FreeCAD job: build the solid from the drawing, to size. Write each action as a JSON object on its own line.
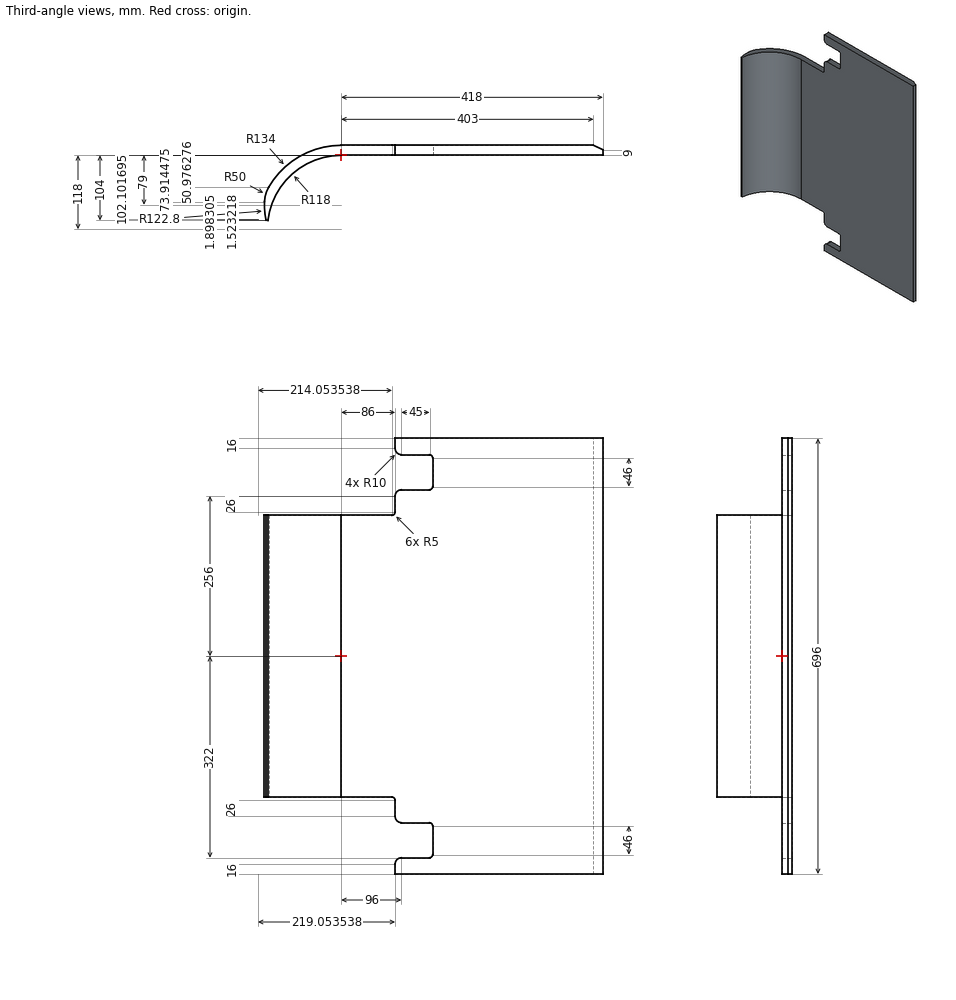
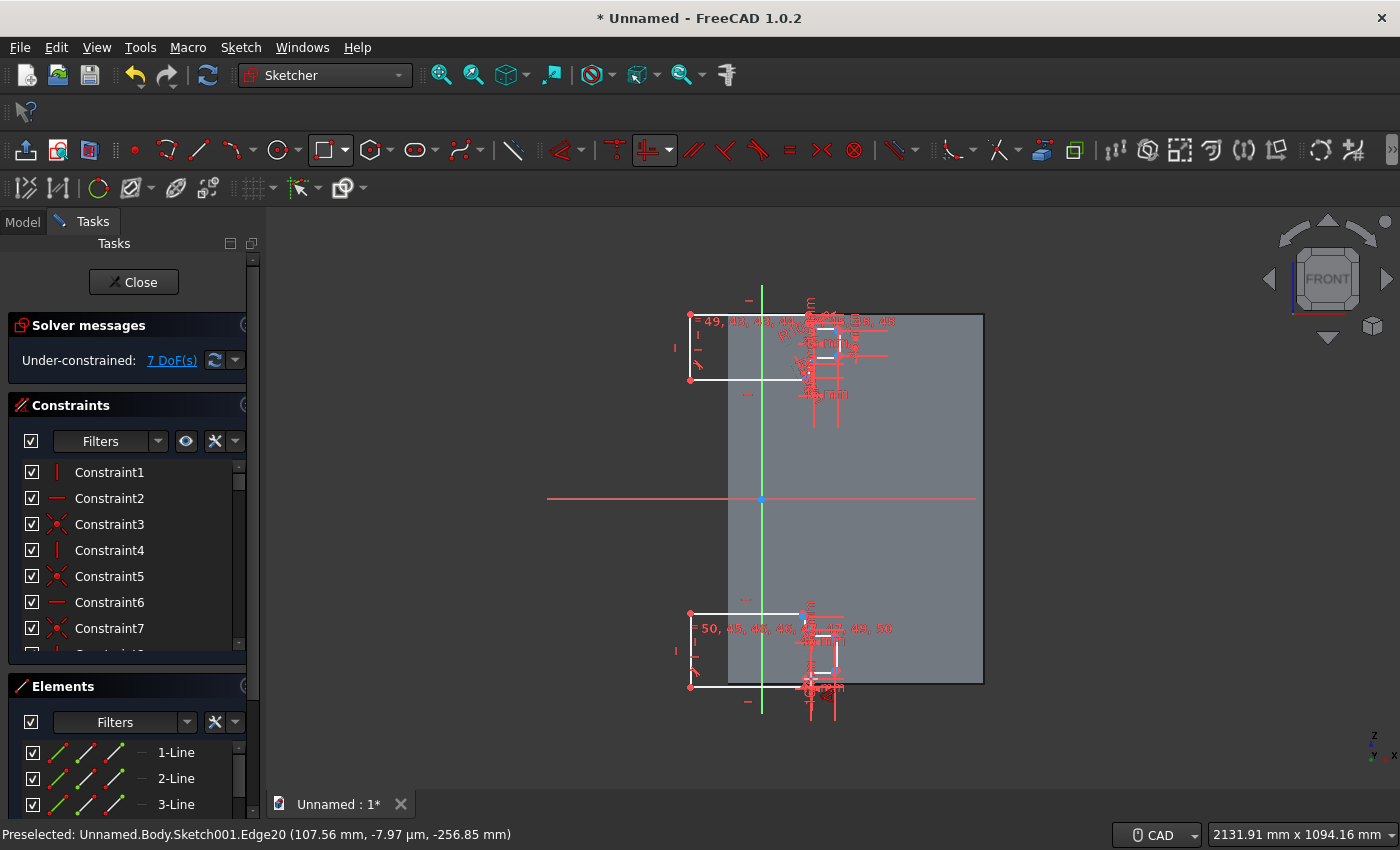
{"action": "scroll", "coordinate": [837, 648], "scroll_direction": "up", "scroll_amount": 3}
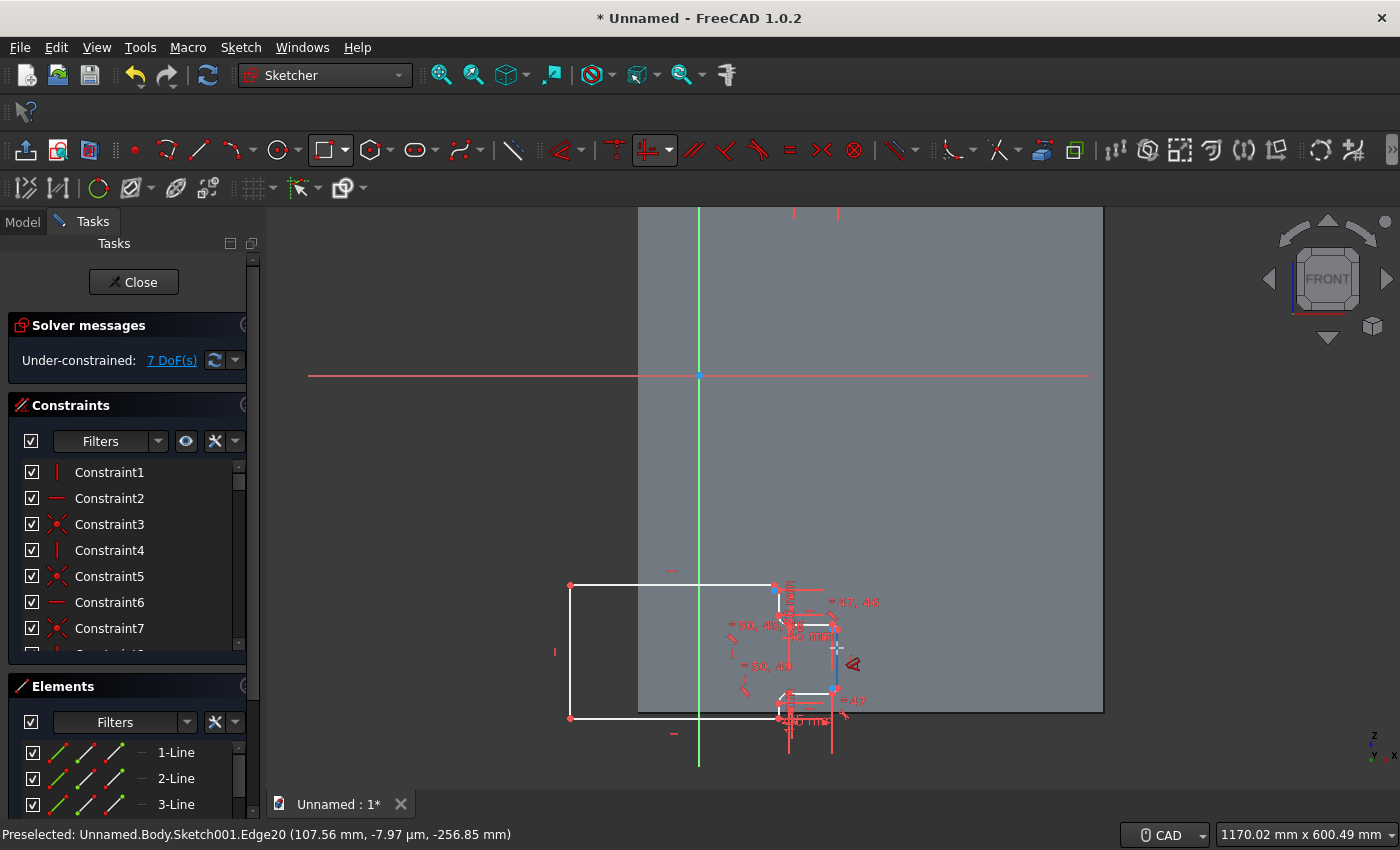
{"action": "left_click", "coordinate": [837, 647]}
{"action": "left_click", "coordinate": [871, 659]}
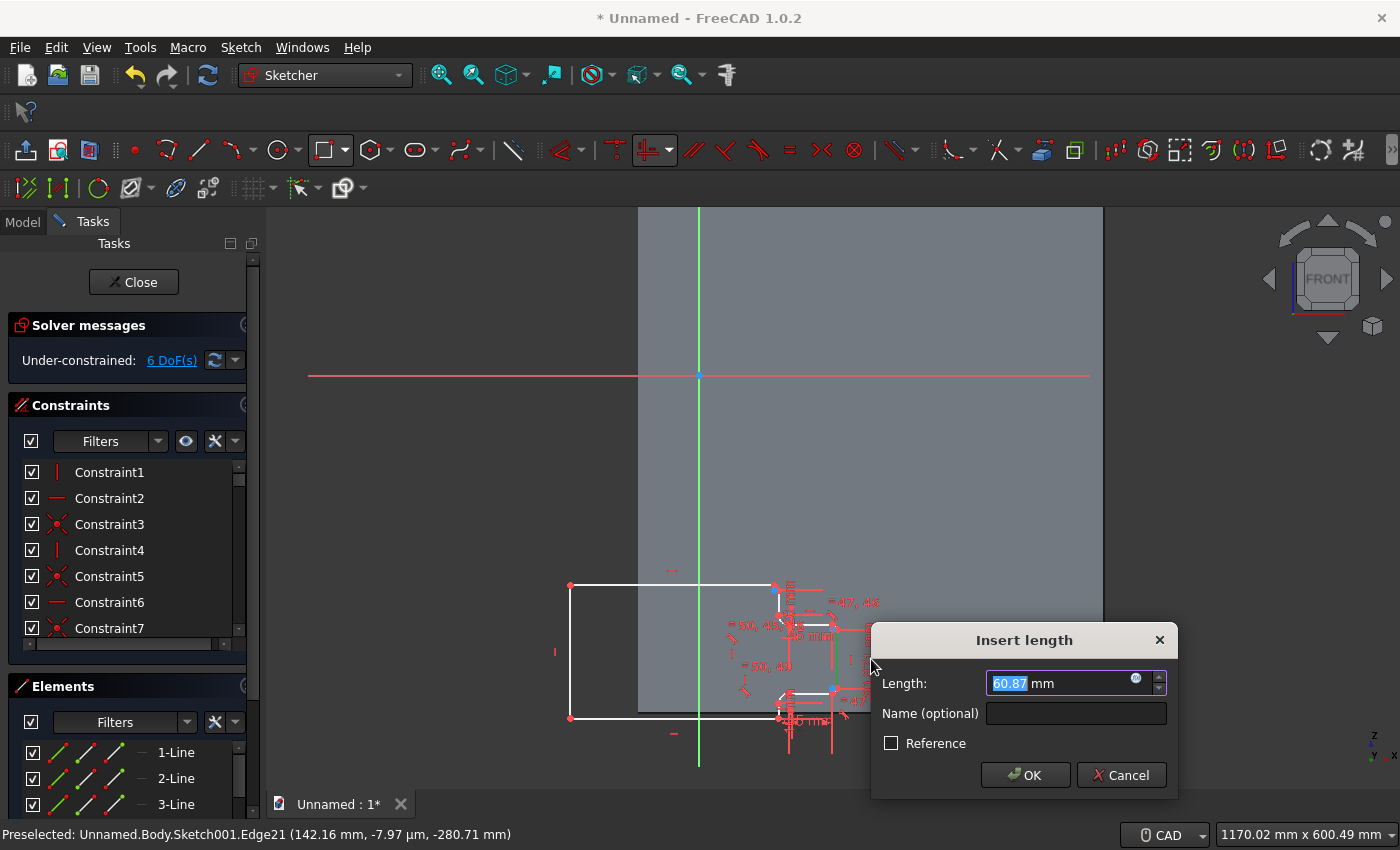
{"action": "type", "text": "46"}
{"action": "key", "text": "Return"}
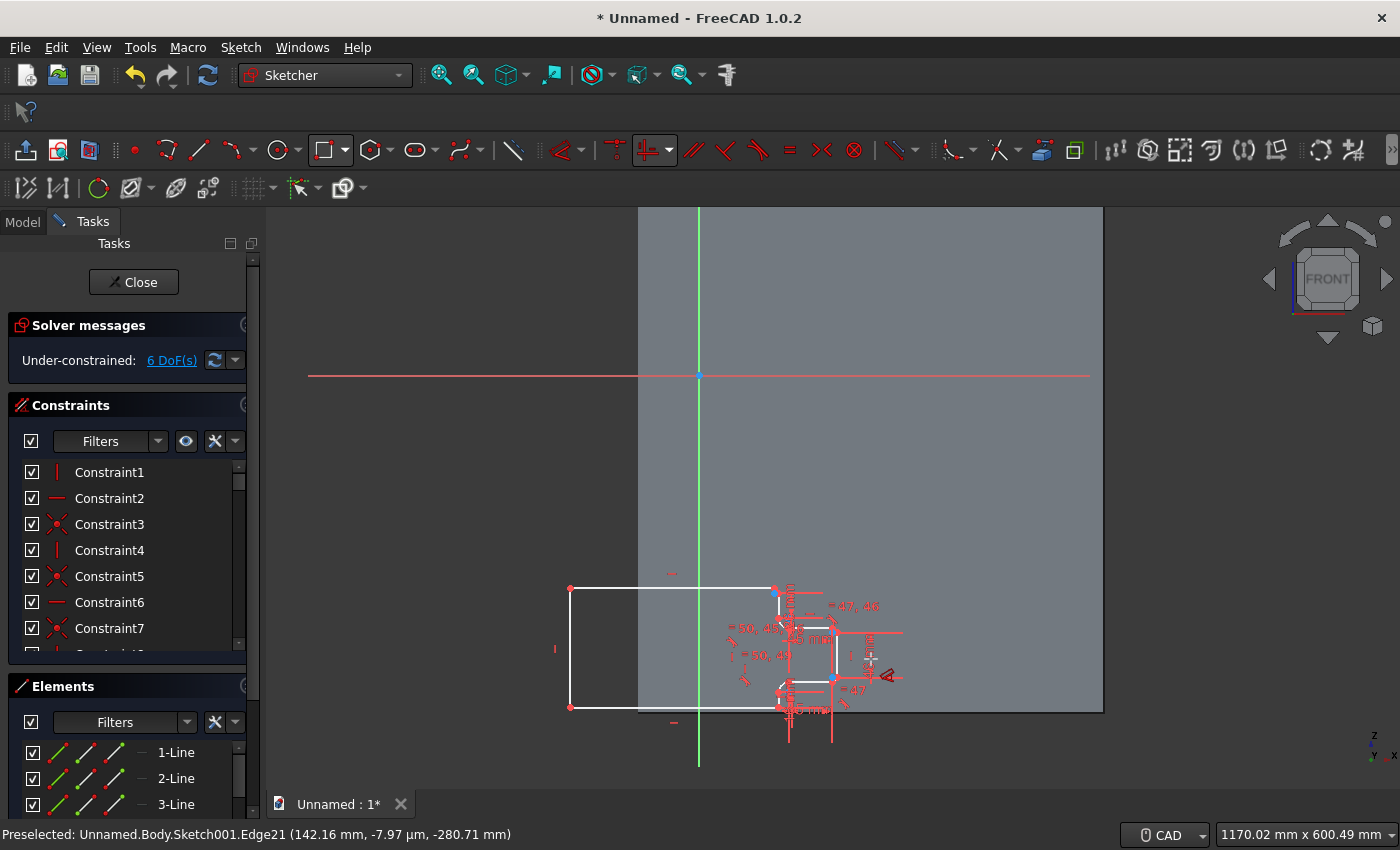
{"action": "scroll", "coordinate": [836, 646], "scroll_direction": "down", "scroll_amount": 3}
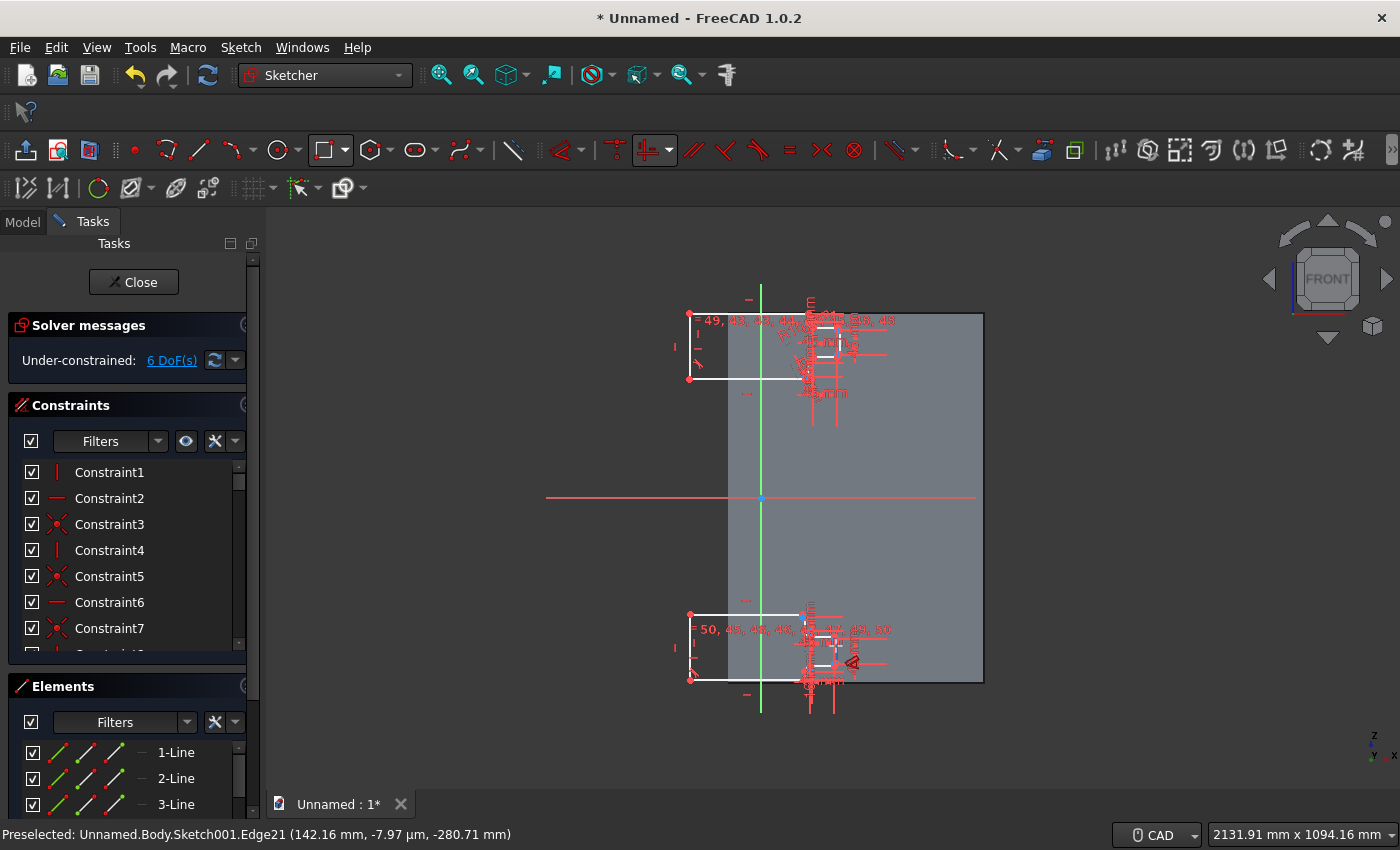
{"action": "scroll", "coordinate": [808, 363], "scroll_direction": "up", "scroll_amount": 5}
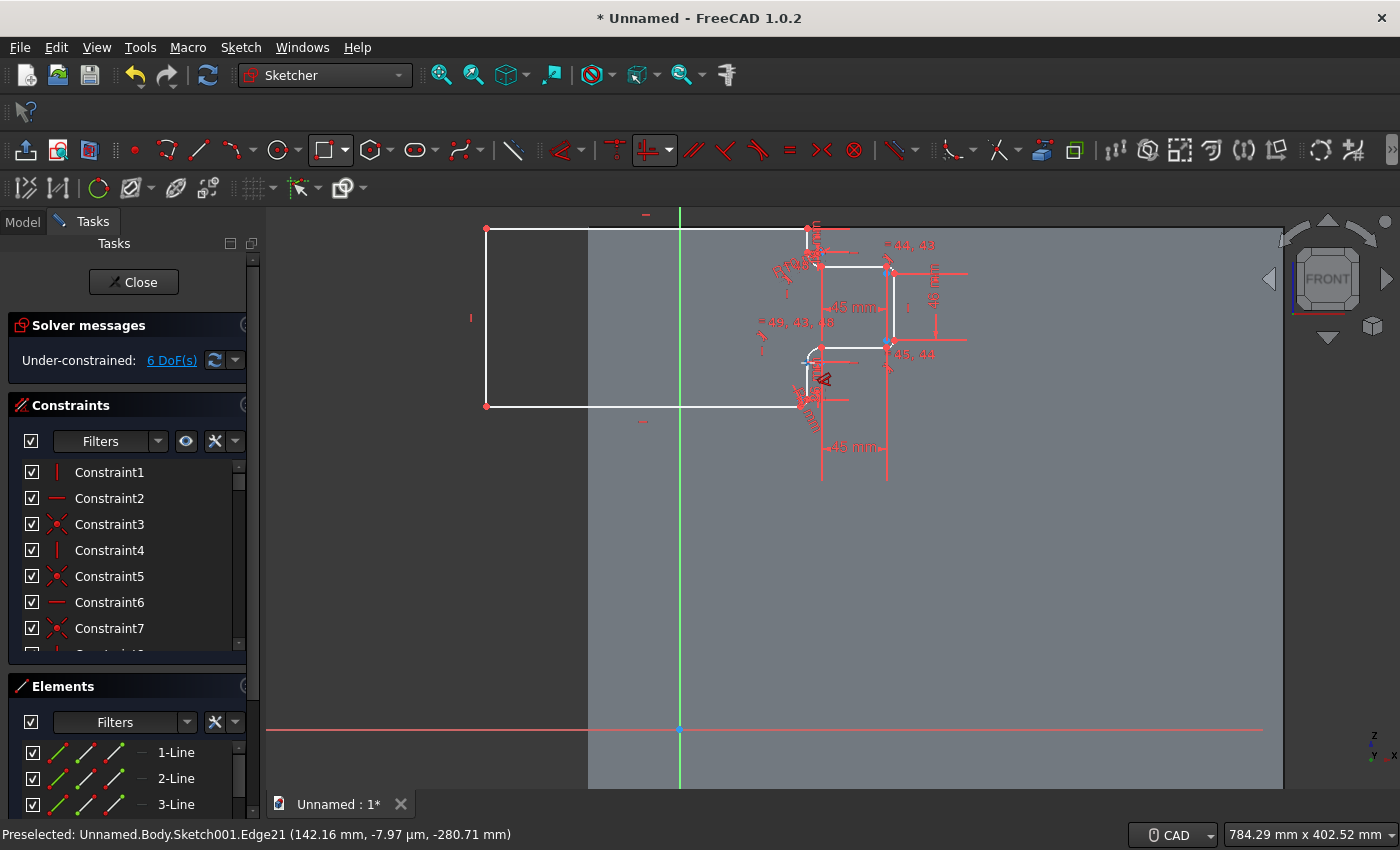
{"action": "left_click", "coordinate": [807, 362]}
{"action": "left_click", "coordinate": [744, 328]}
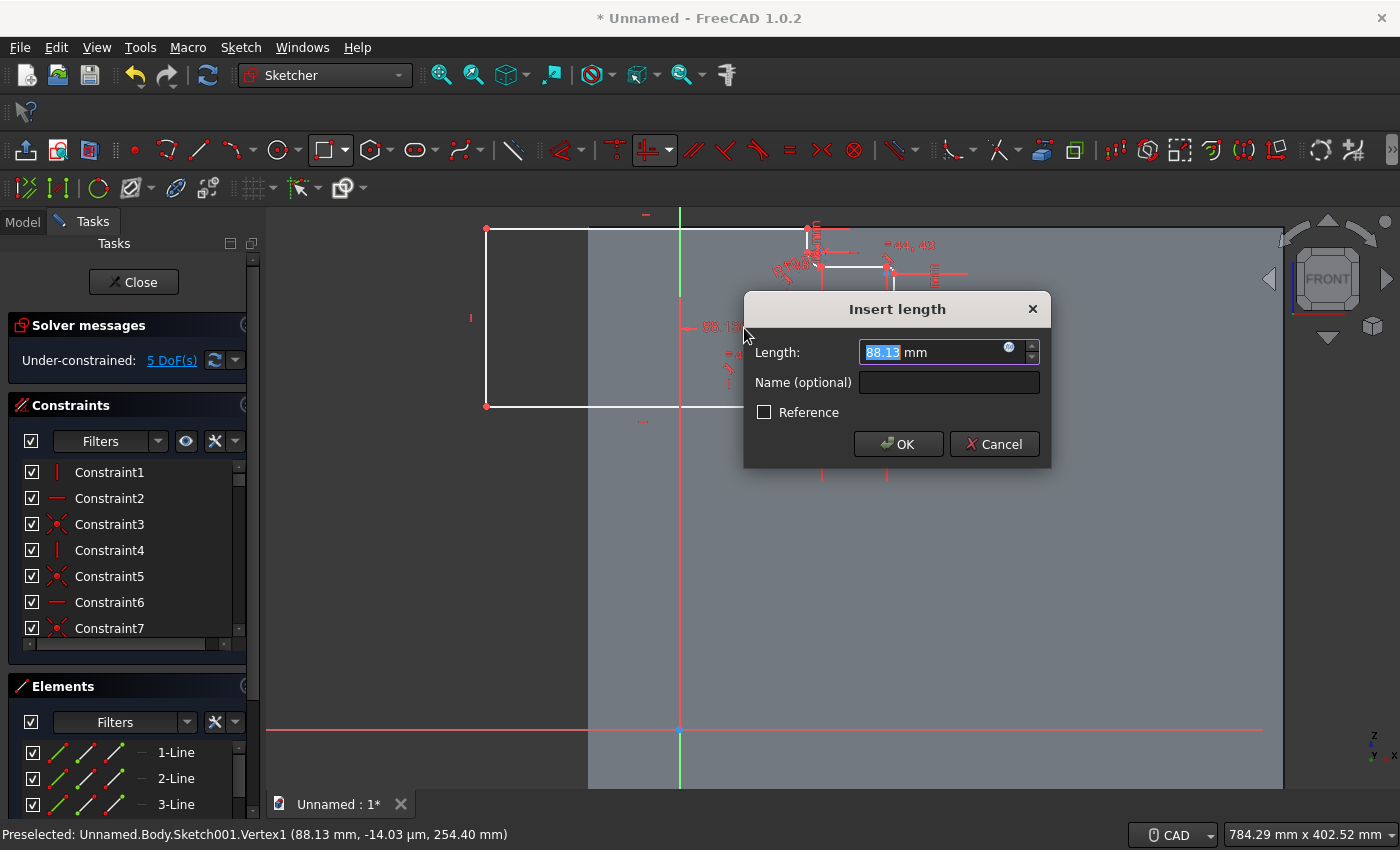
{"action": "type", "text": "86"}
{"action": "key", "text": "Return"}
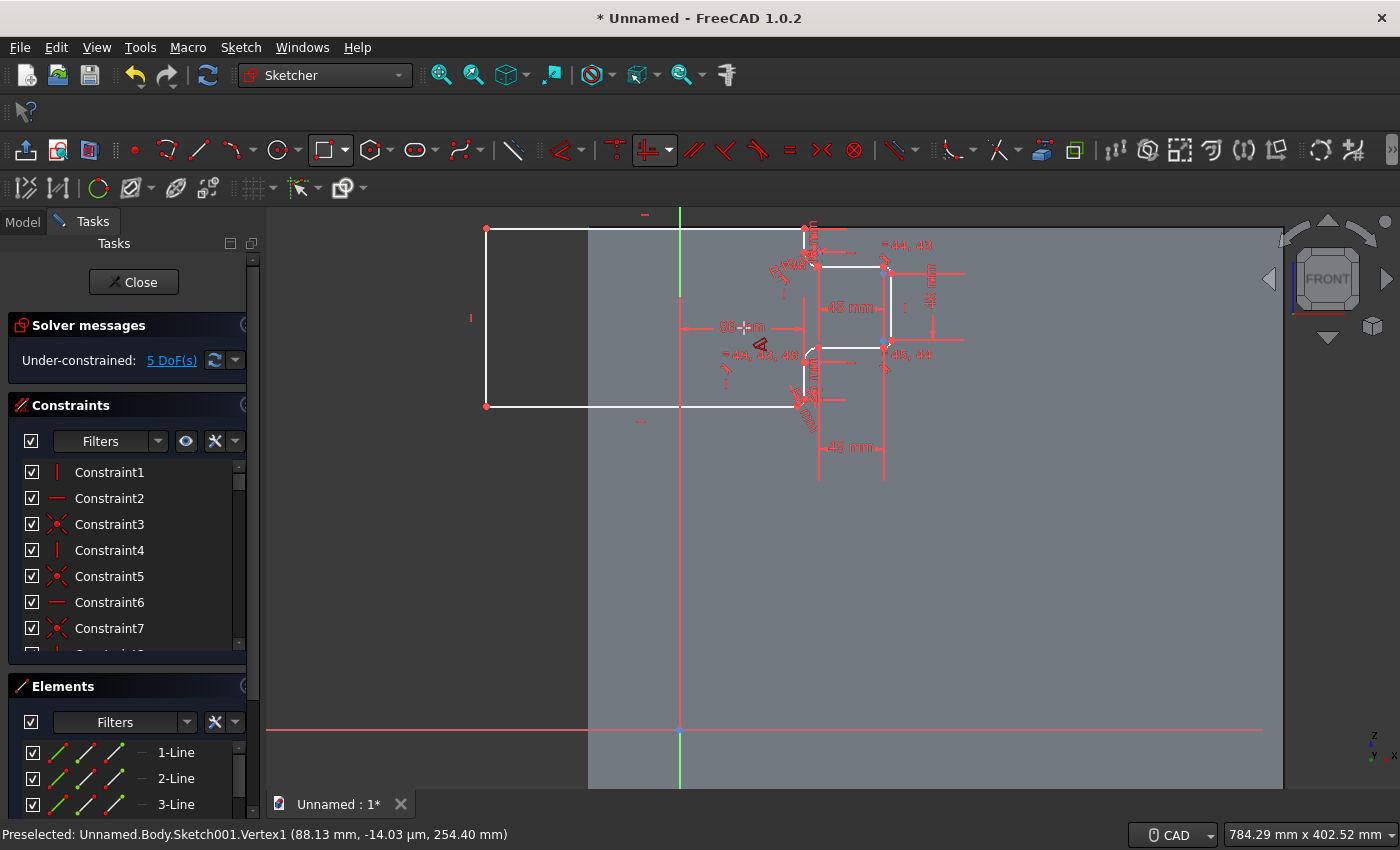
{"action": "scroll", "coordinate": [808, 363], "scroll_direction": "down", "scroll_amount": 5}